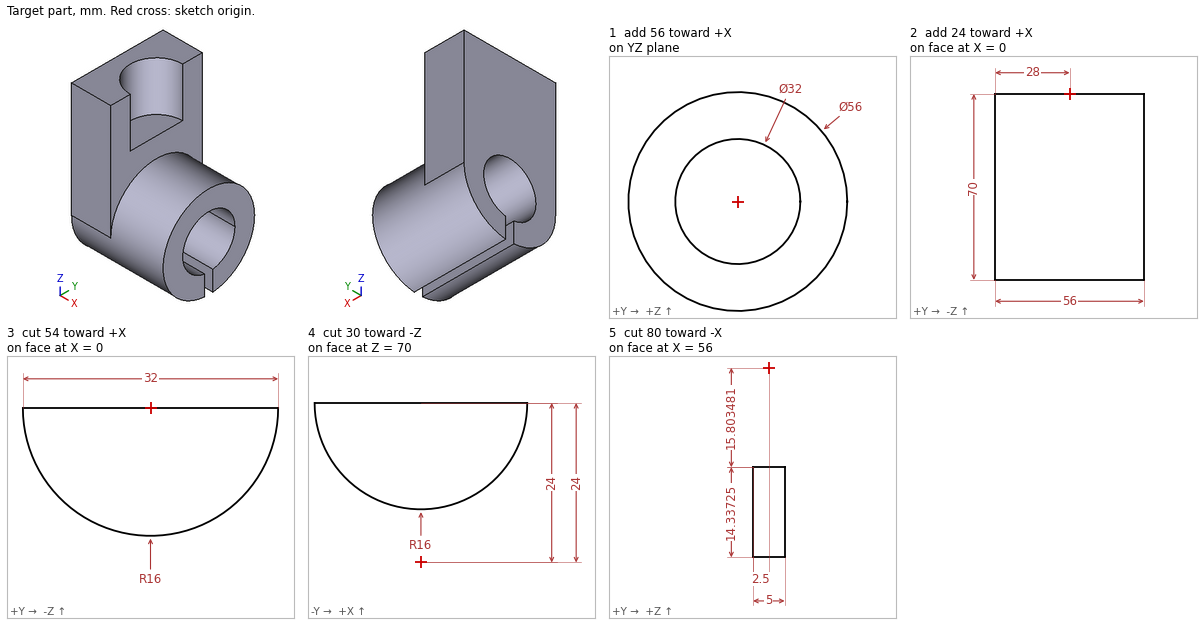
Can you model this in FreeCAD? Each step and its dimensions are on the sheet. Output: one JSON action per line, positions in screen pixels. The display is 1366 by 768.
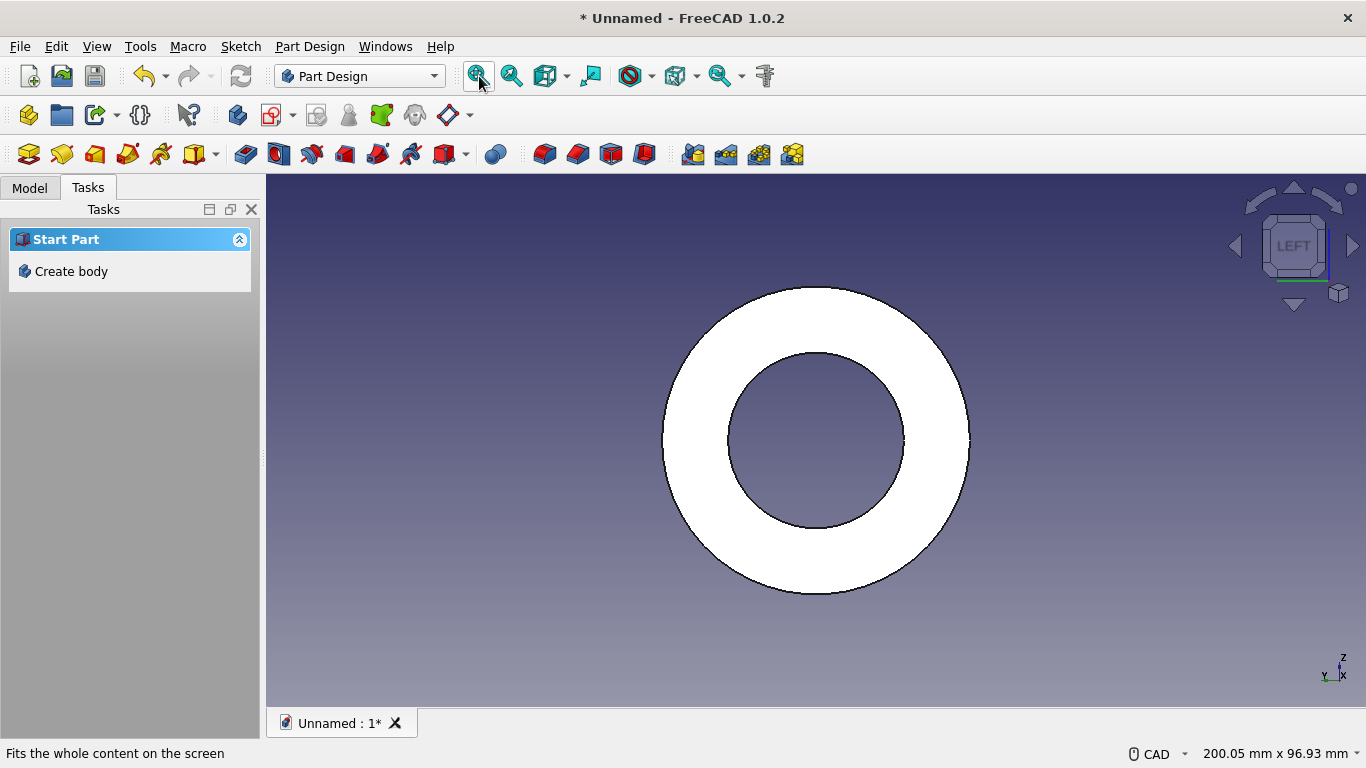
{"action": "left_click", "coordinate": [728, 527]}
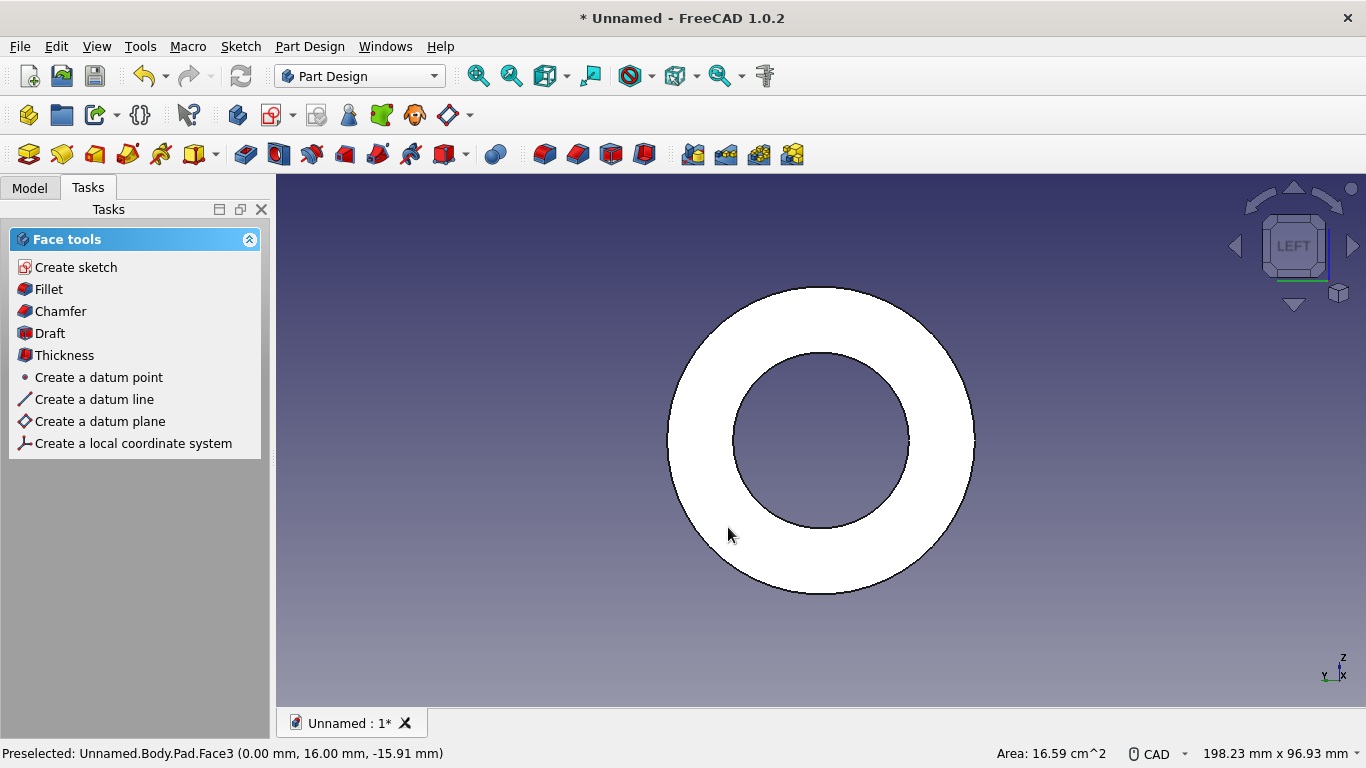
{"action": "left_click", "coordinate": [270, 116]}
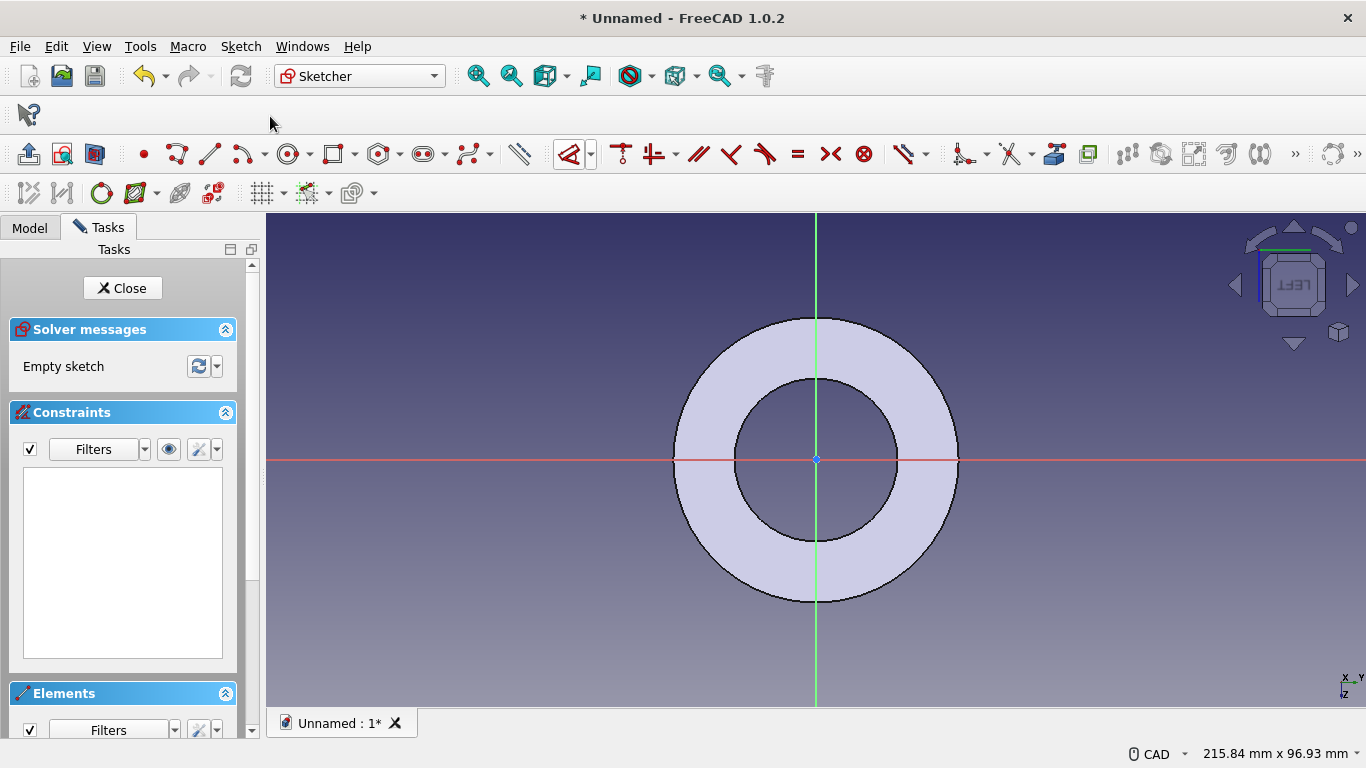
{"action": "scroll", "coordinate": [608, 241], "scroll_direction": "down", "scroll_amount": 2}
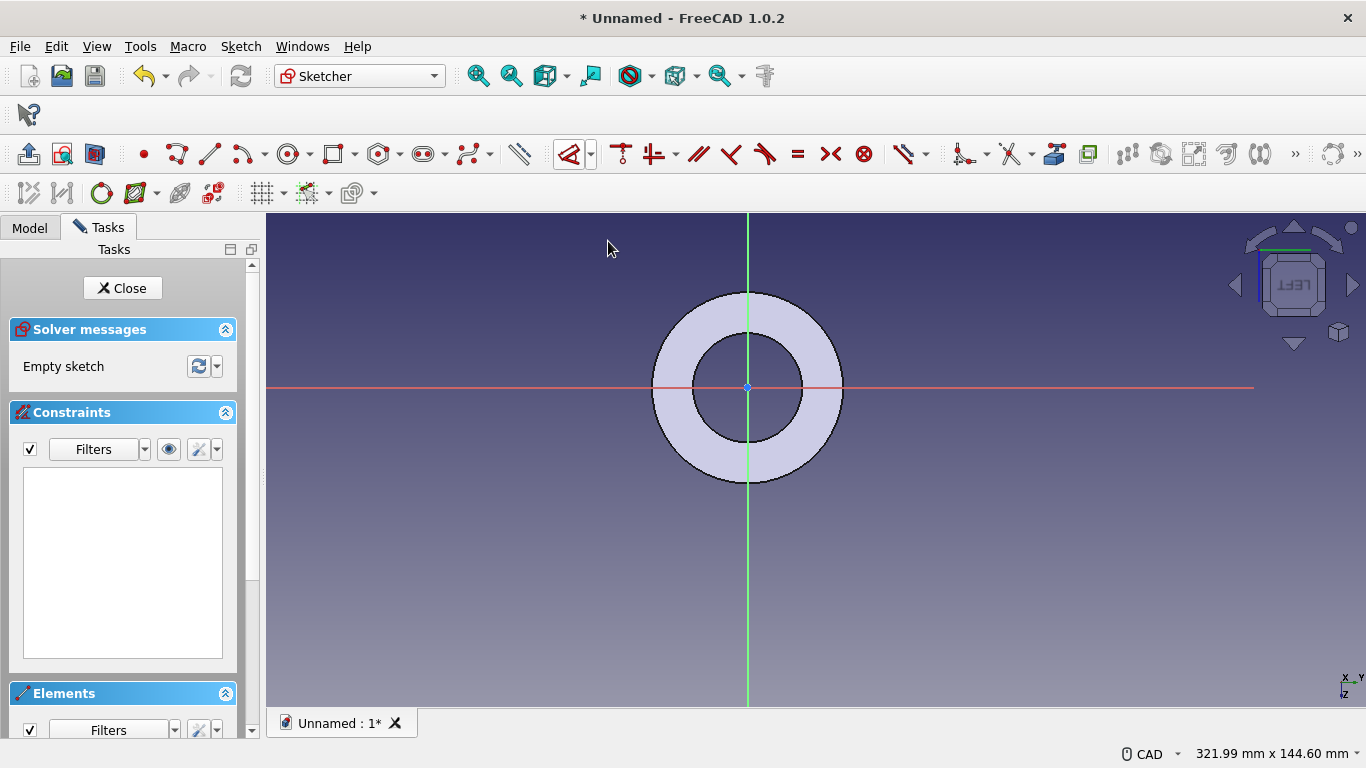
{"action": "left_click", "coordinate": [332, 154]}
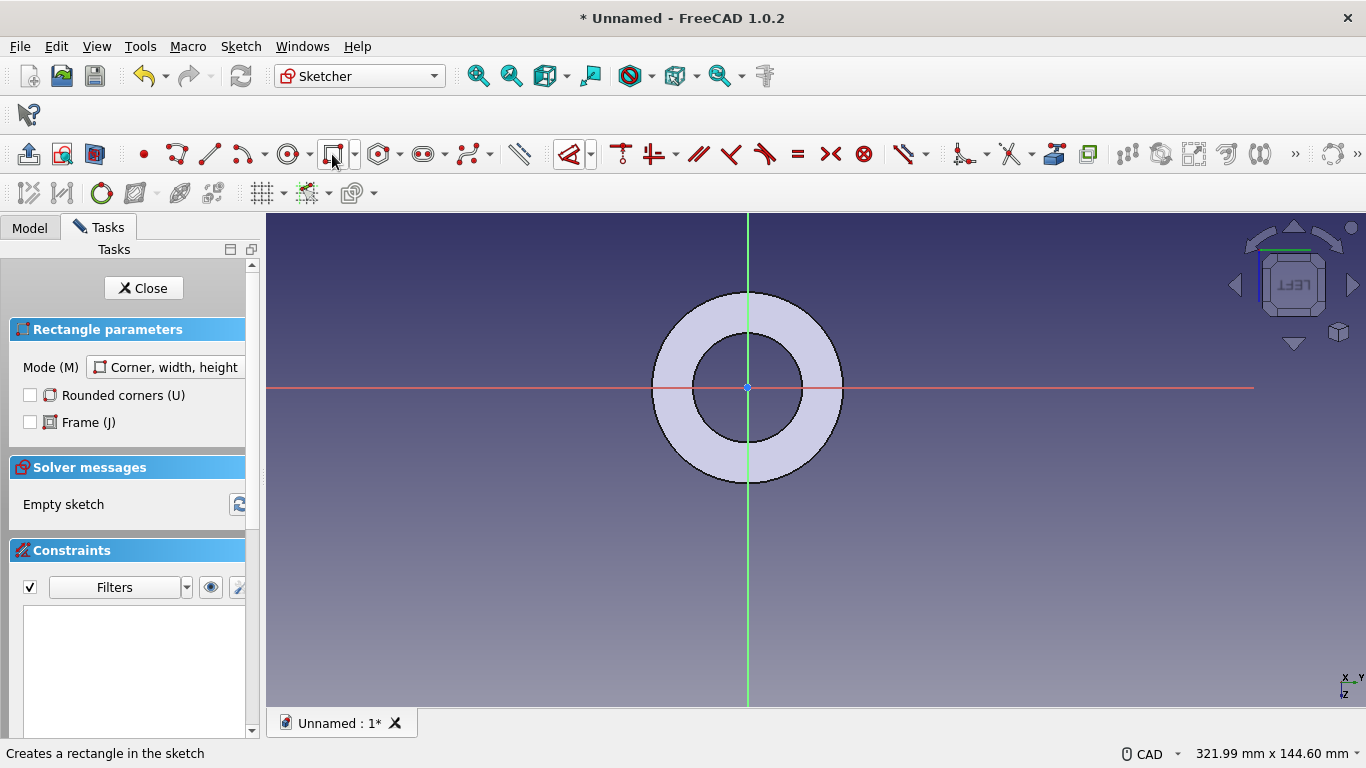
{"action": "left_click", "coordinate": [652, 388]}
{"action": "left_click", "coordinate": [843, 627]}
{"action": "key", "text": "Escape"}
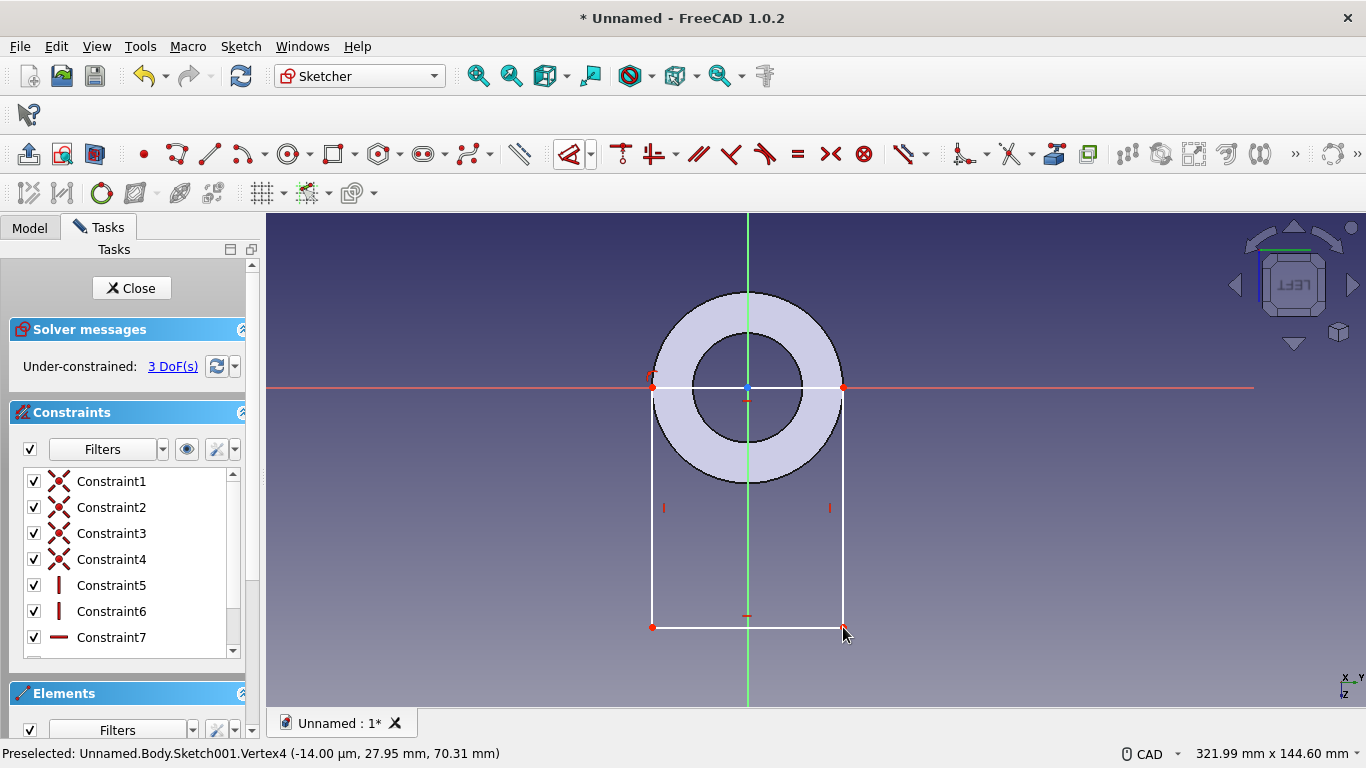
{"action": "left_click", "coordinate": [652, 460]}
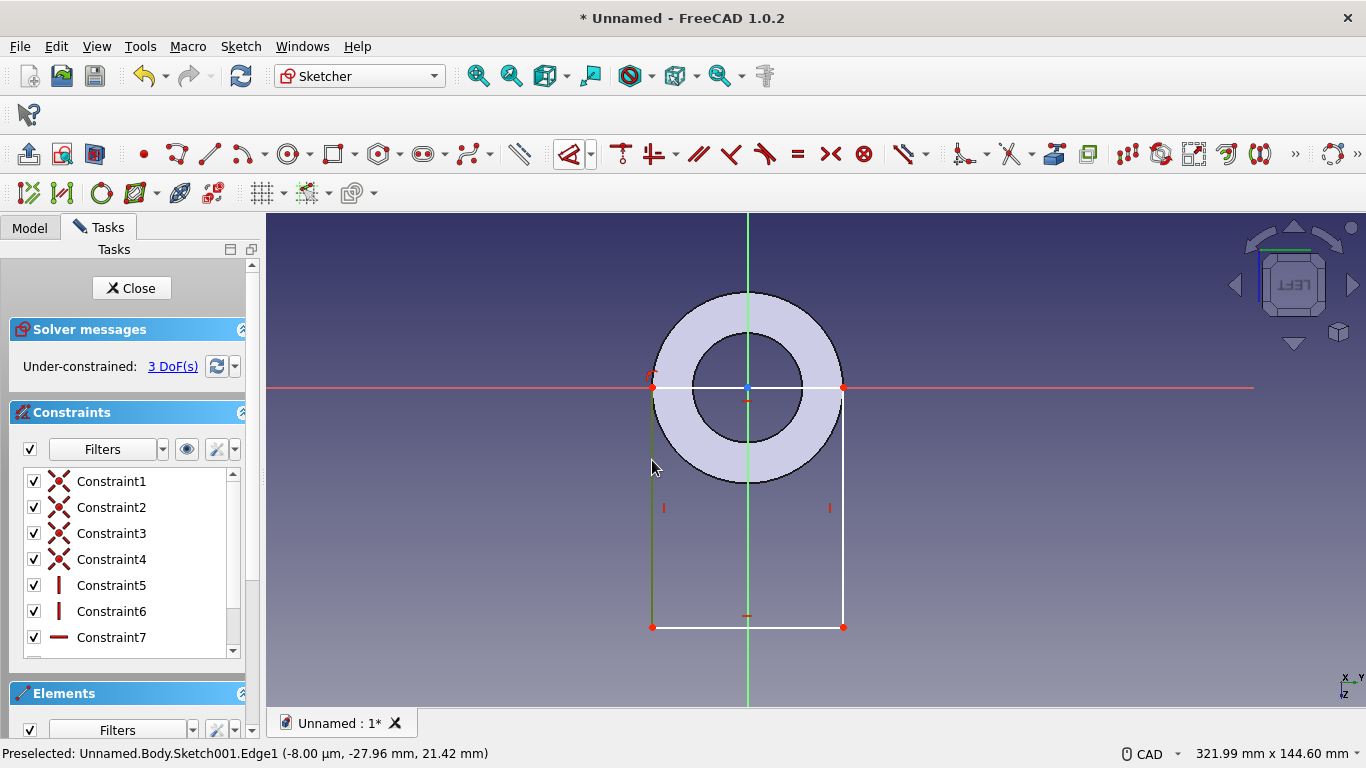
{"action": "left_click", "coordinate": [590, 154]}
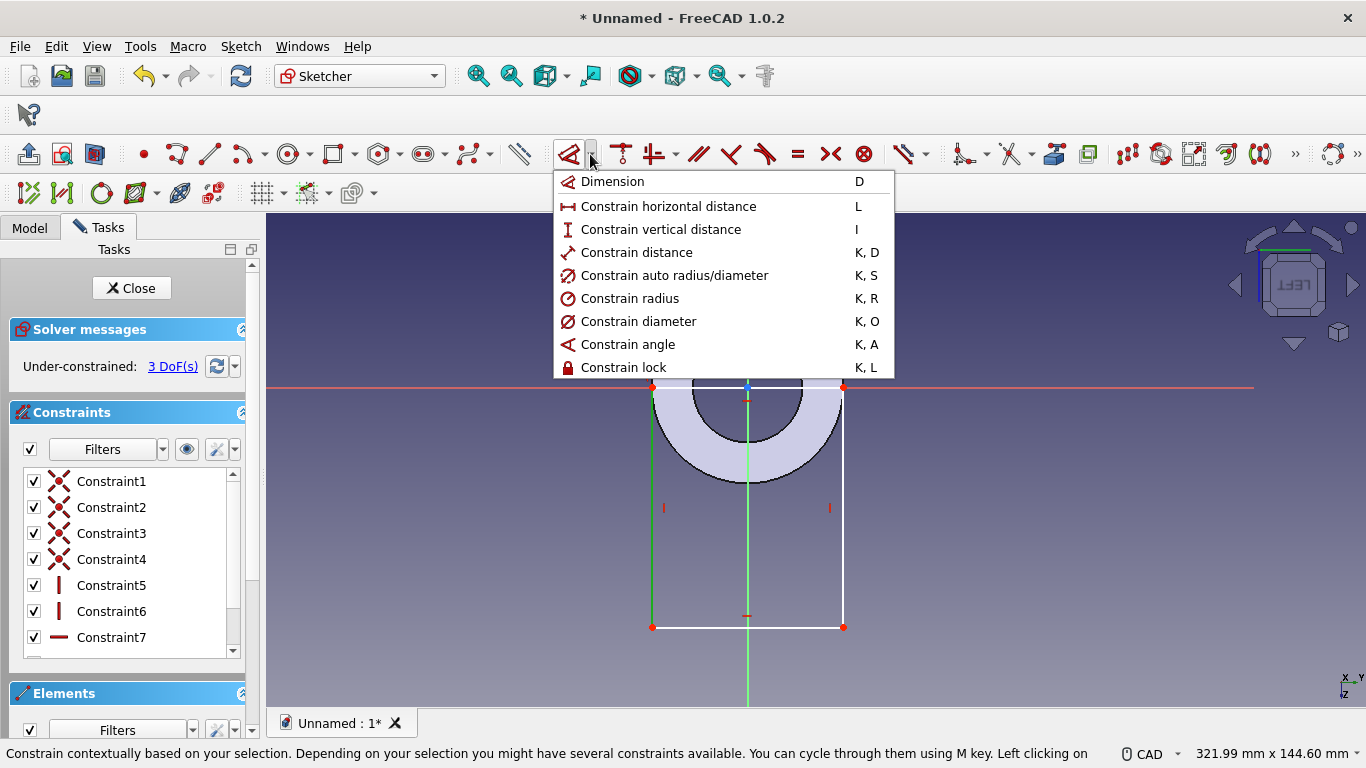
{"action": "left_click", "coordinate": [724, 230]}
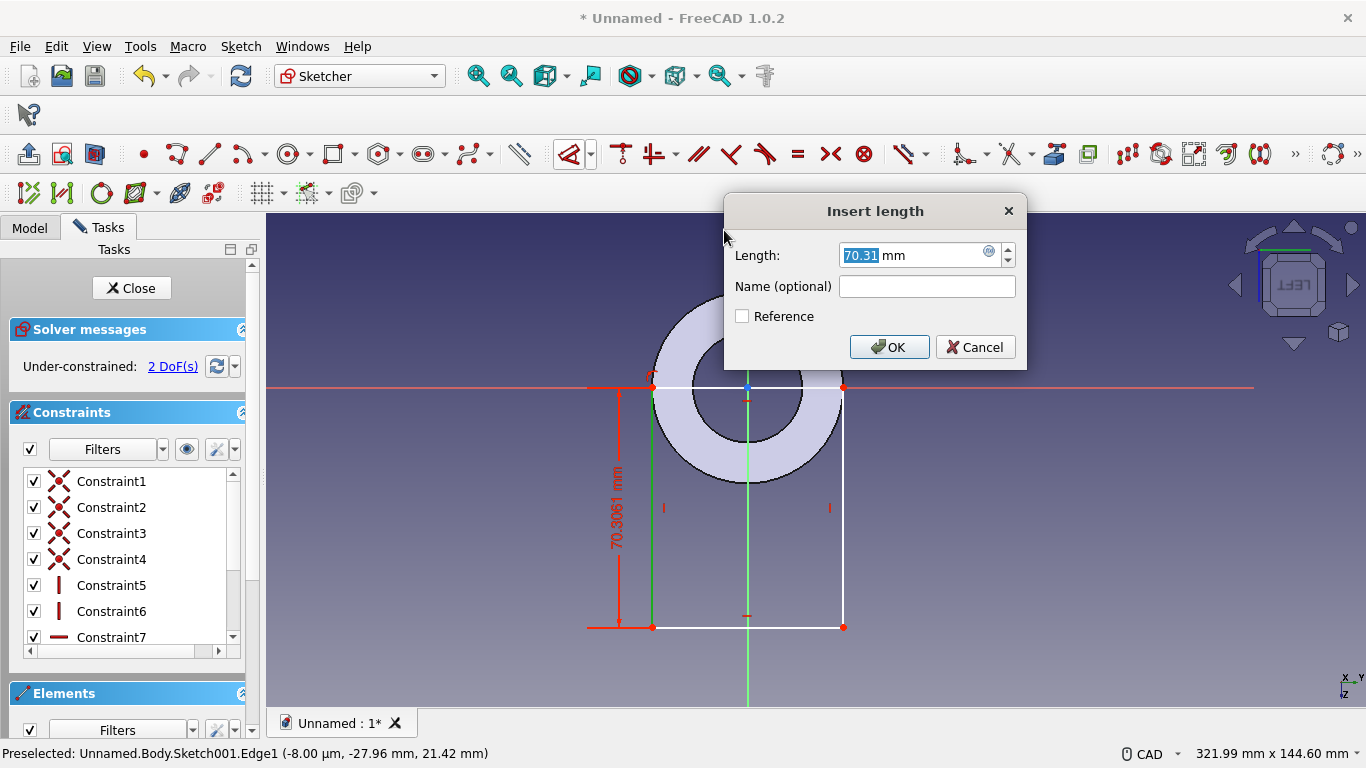
{"action": "type", "text": "70"}
{"action": "key", "text": "Return"}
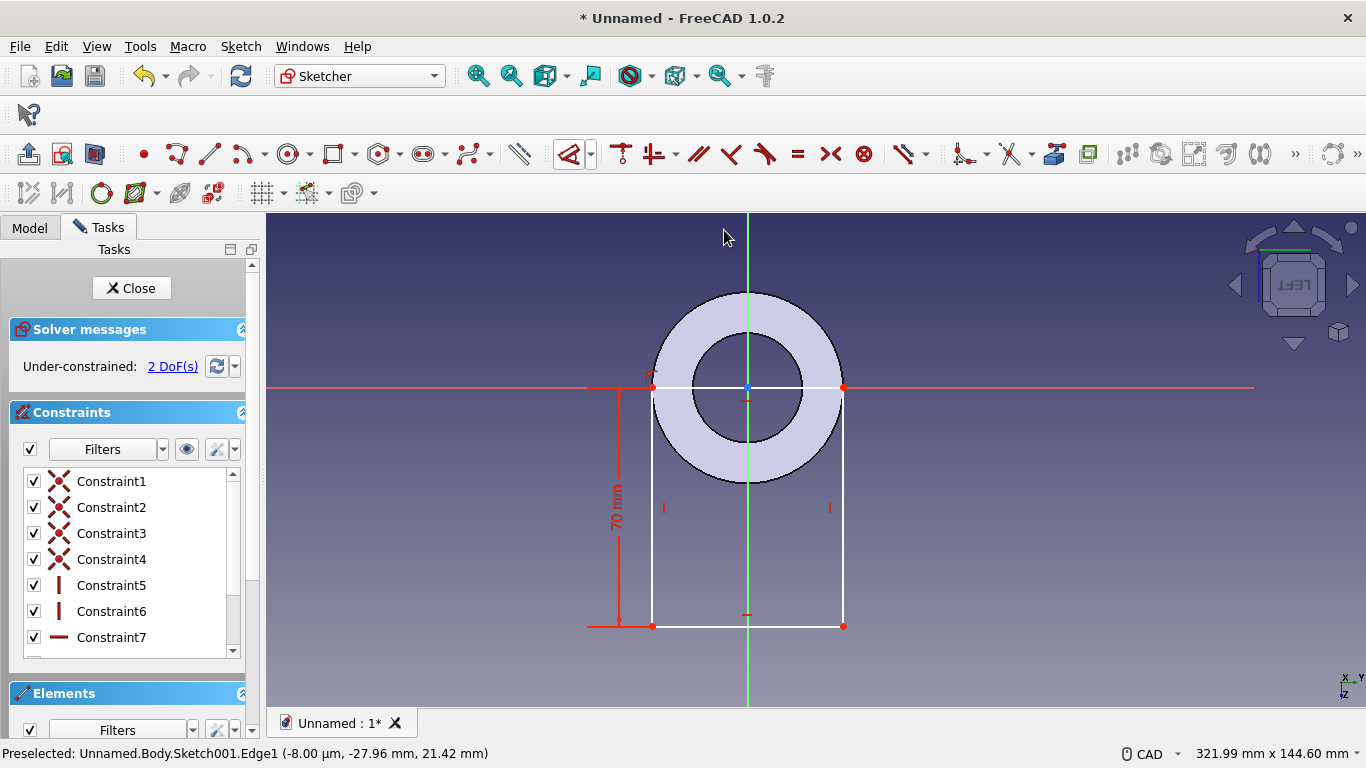
{"action": "left_click", "coordinate": [709, 627]}